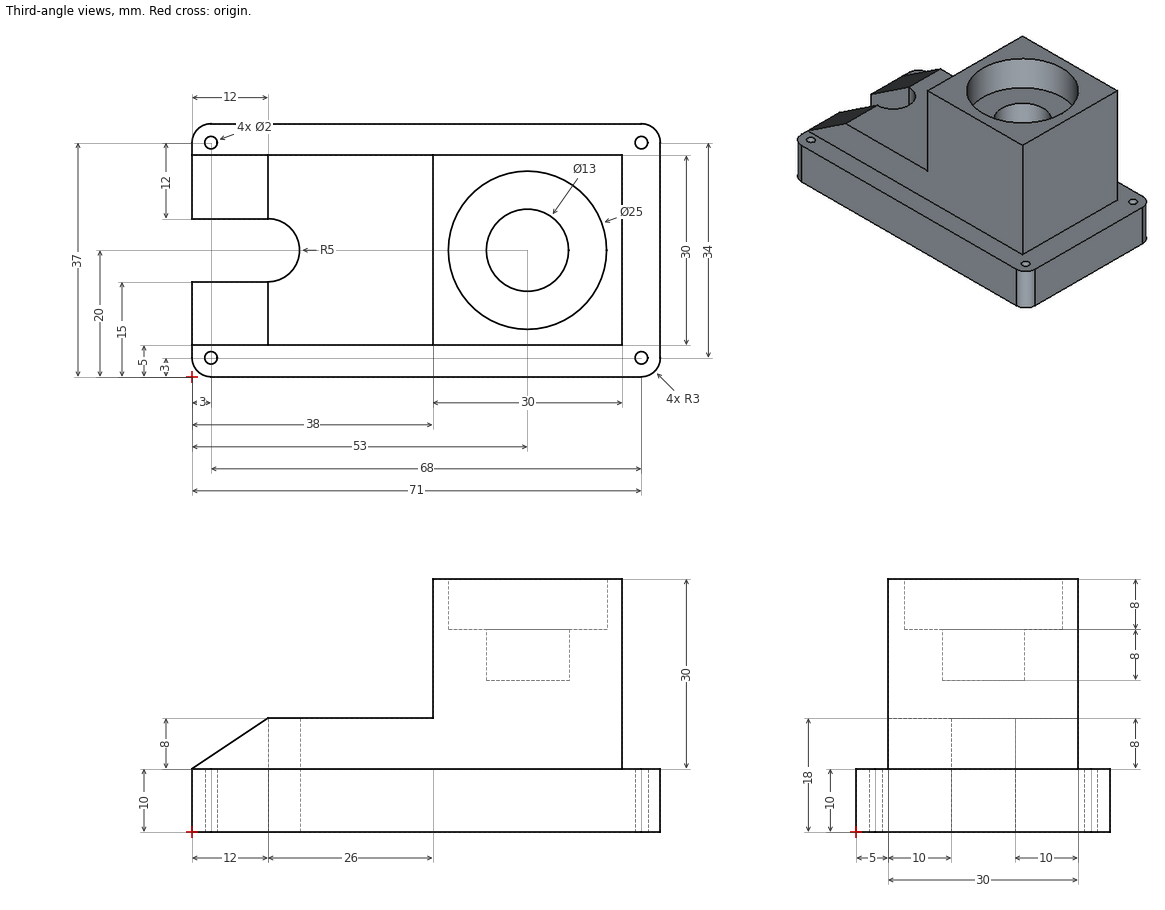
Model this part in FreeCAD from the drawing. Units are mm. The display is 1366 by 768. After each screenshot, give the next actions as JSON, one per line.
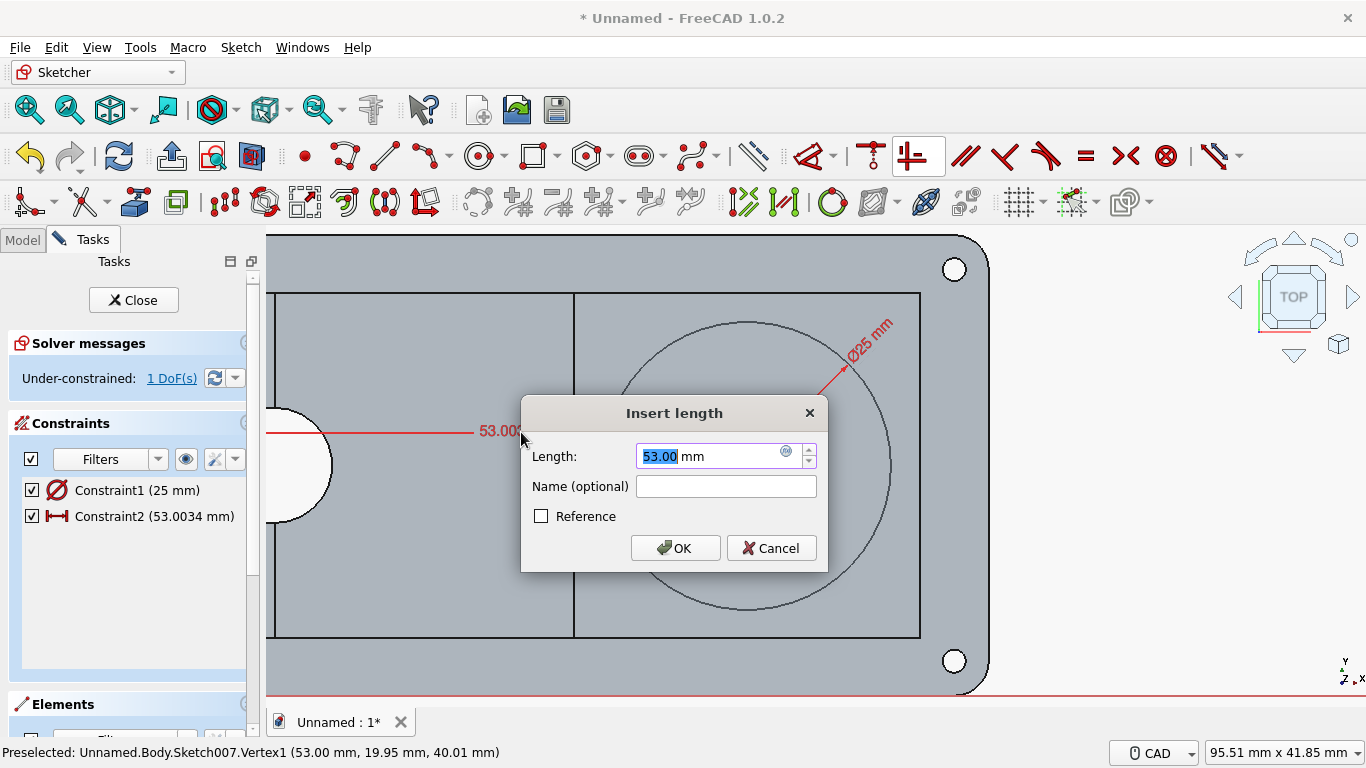
{"action": "type", "text": "53"}
{"action": "key", "text": "Return"}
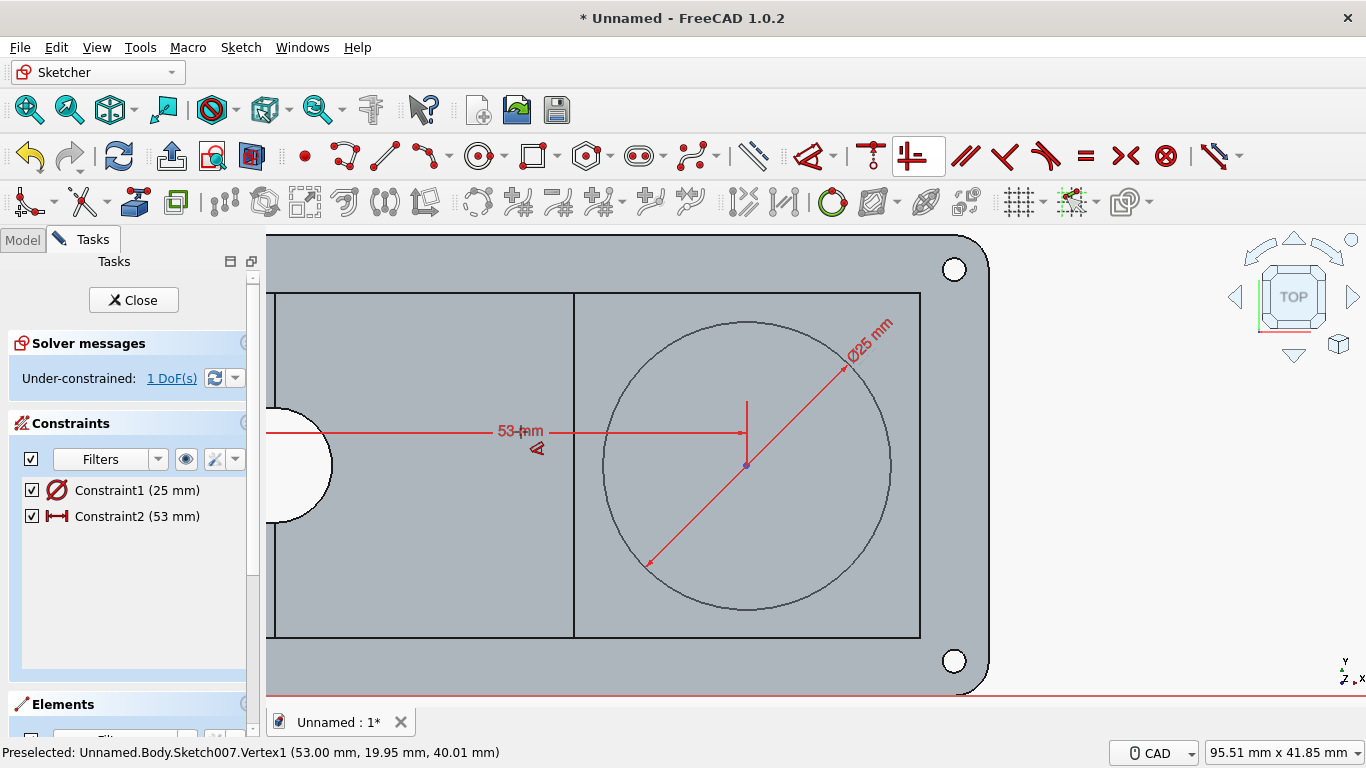
{"action": "left_click", "coordinate": [747, 466]}
{"action": "left_click", "coordinate": [781, 573]}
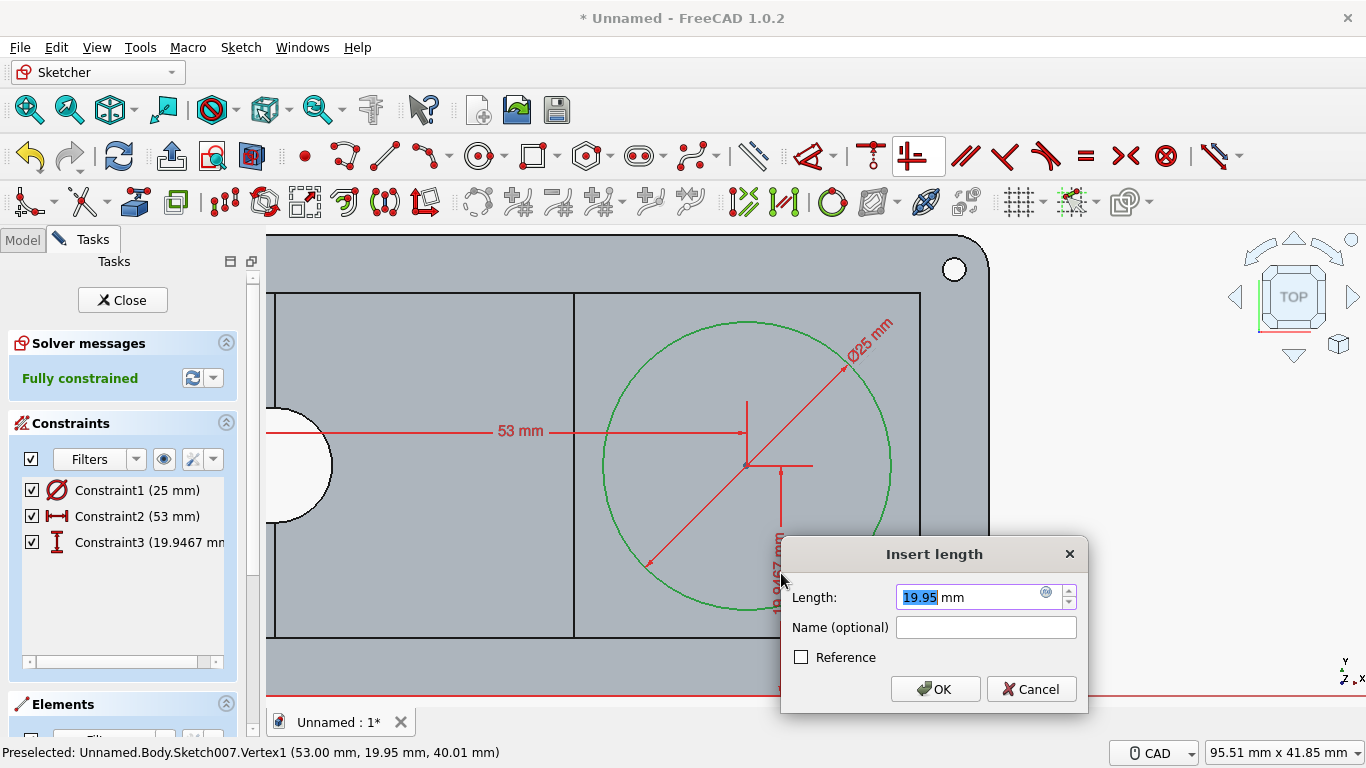
{"action": "type", "text": "20"}
{"action": "key", "text": "Return"}
{"action": "key", "text": "Escape"}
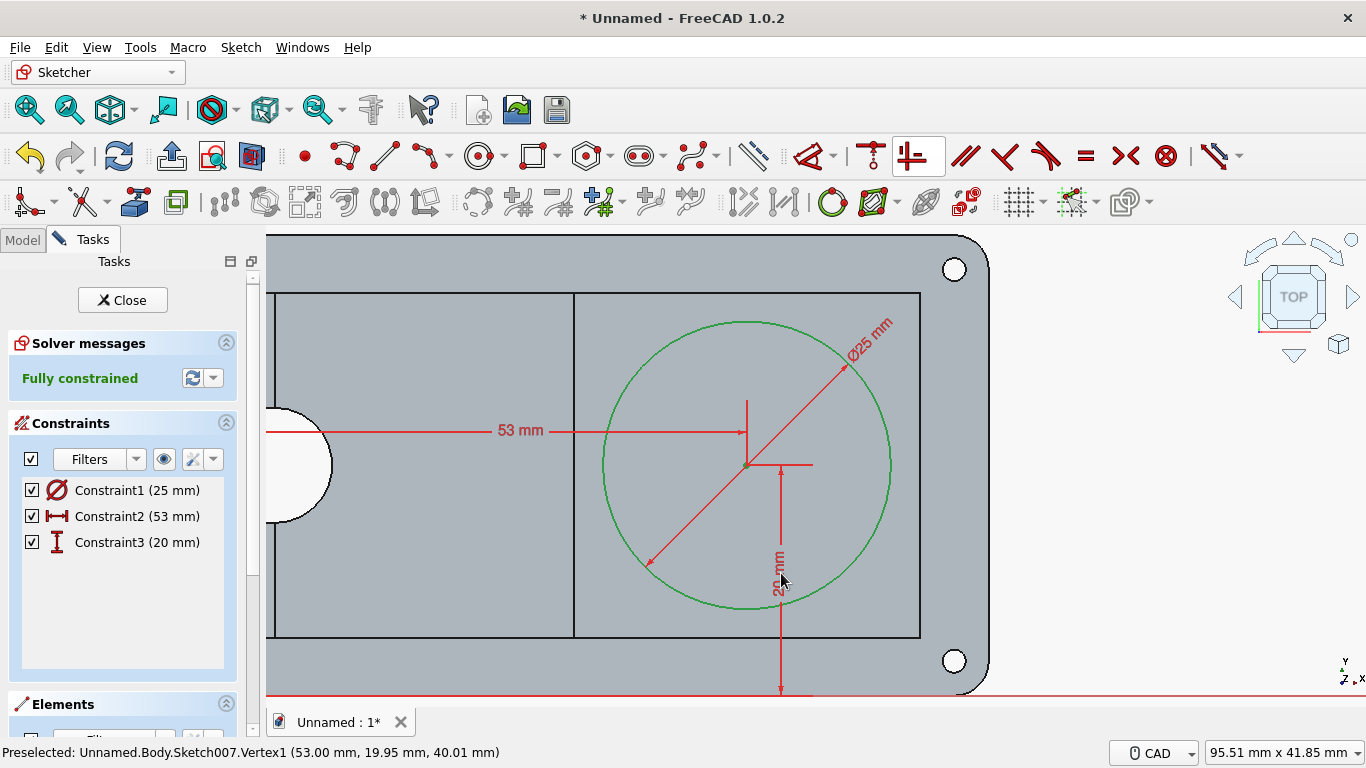
{"action": "left_click", "coordinate": [123, 300]}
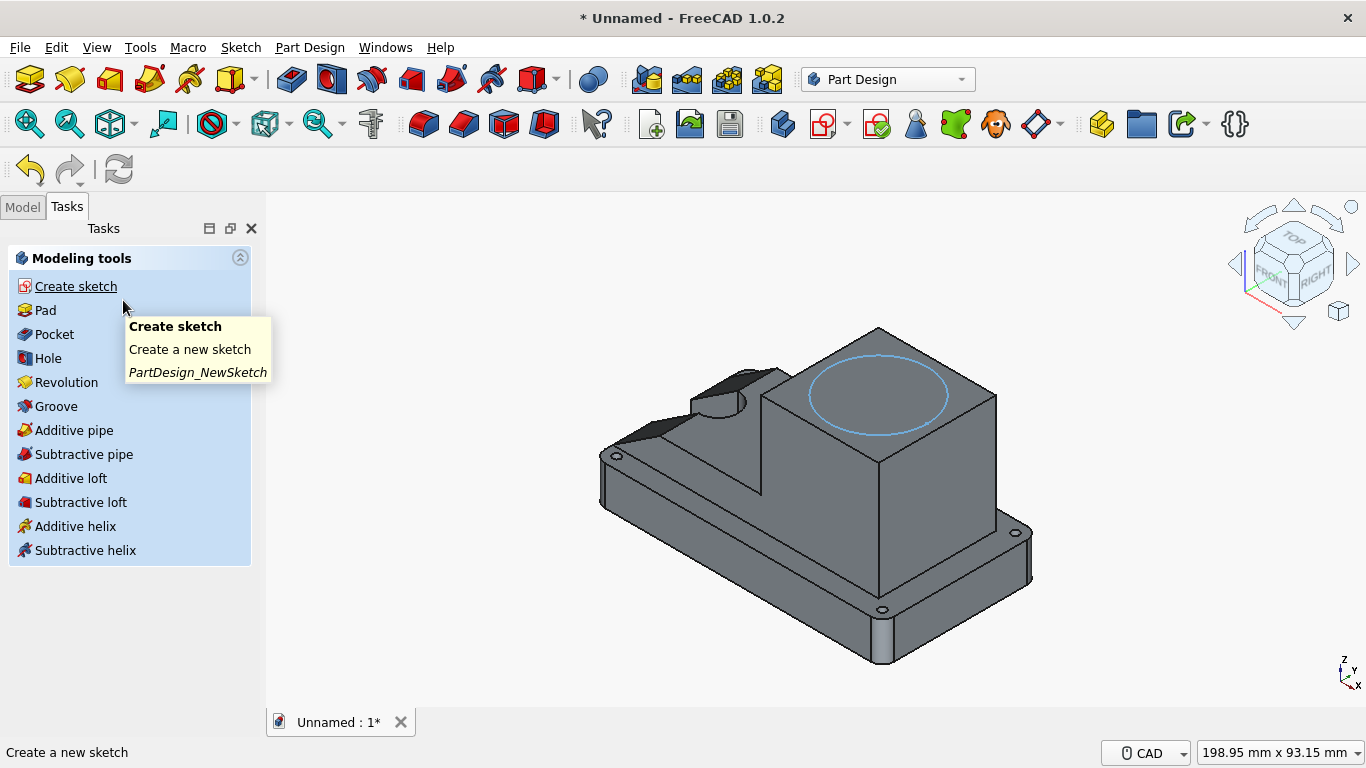
{"action": "left_click", "coordinate": [292, 80]}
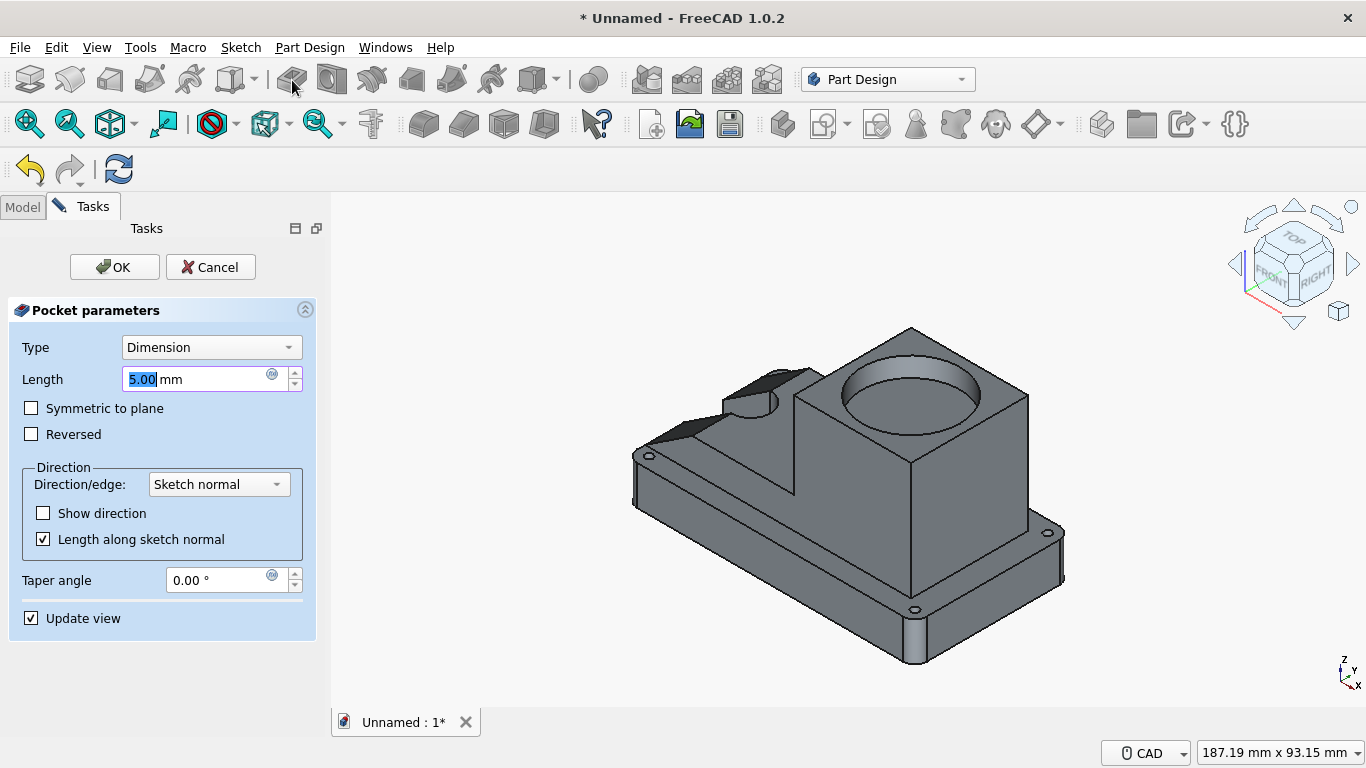
{"action": "type", "text": "8"}
{"action": "key", "text": "Tab"}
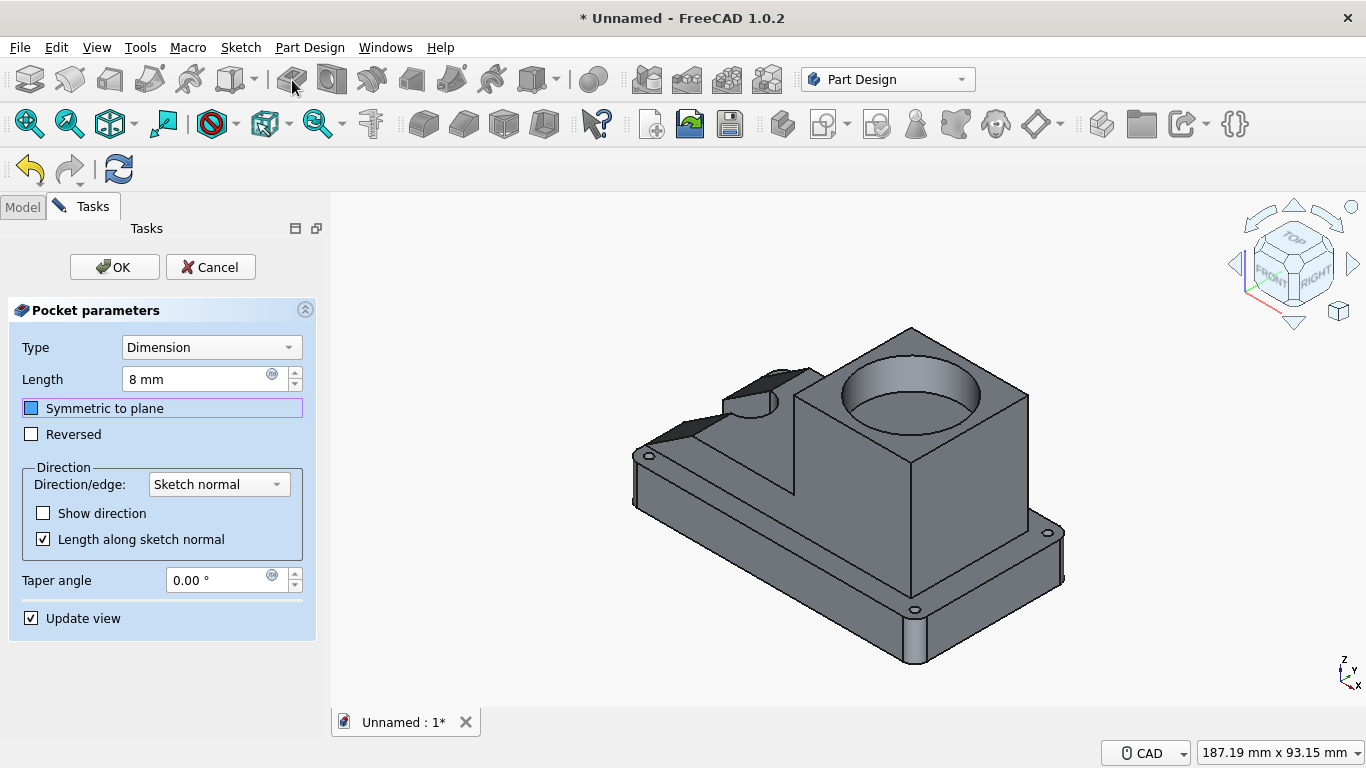
{"action": "left_click", "coordinate": [115, 267]}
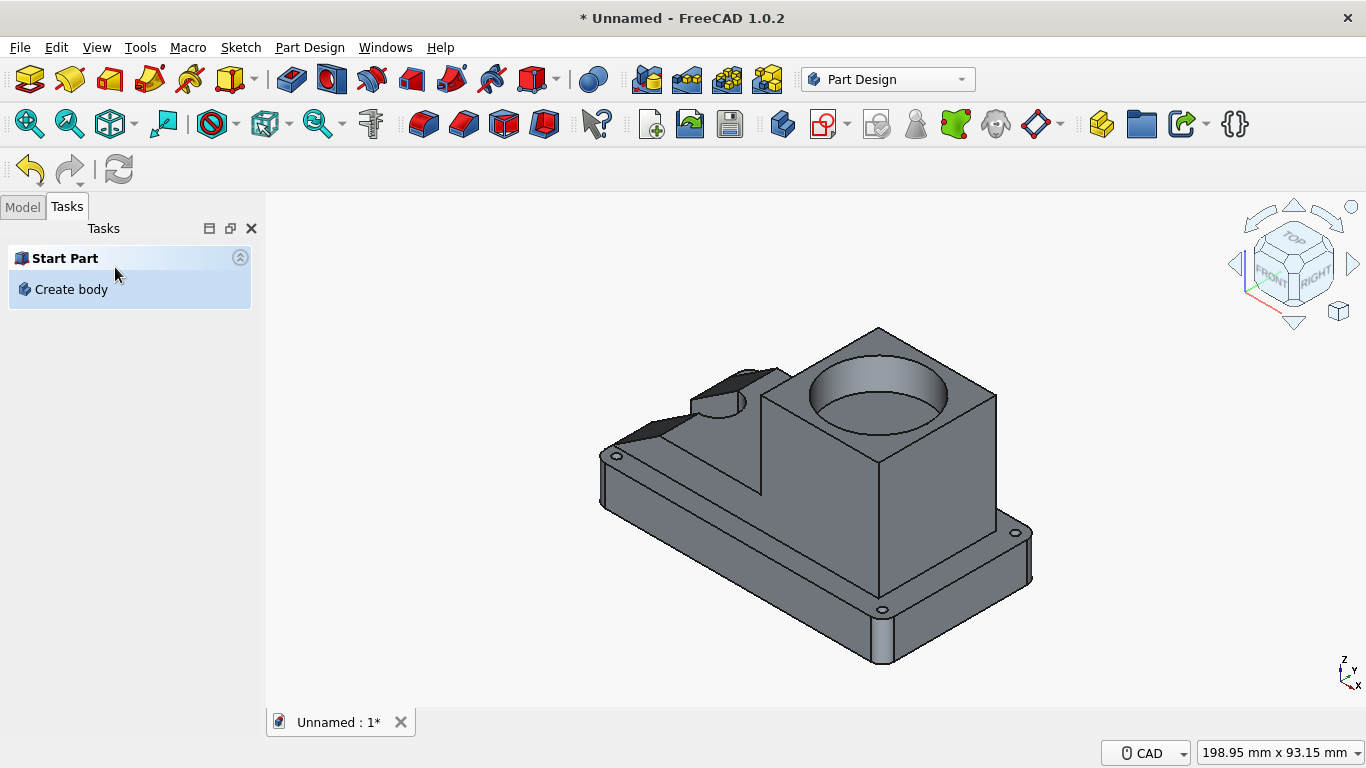
{"action": "left_click", "coordinate": [865, 422]}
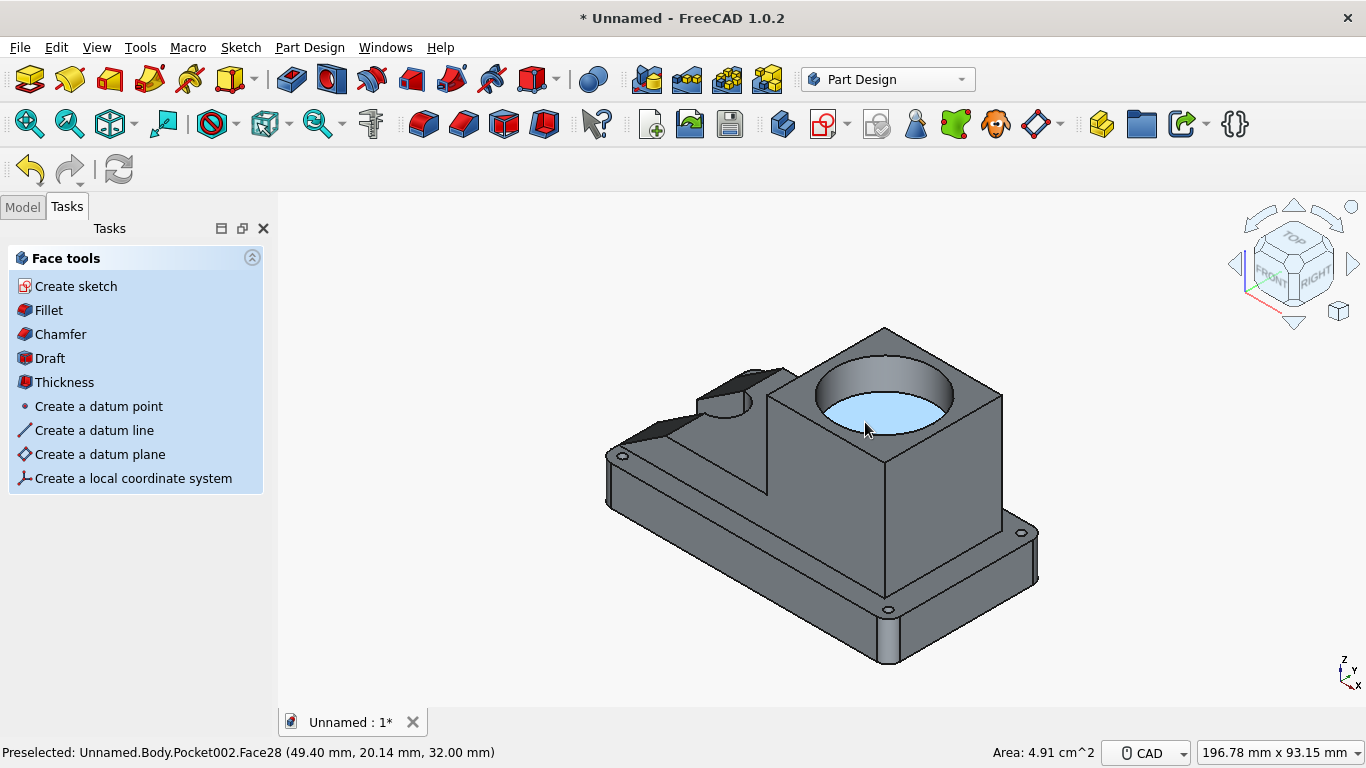
{"action": "left_click", "coordinate": [824, 124]}